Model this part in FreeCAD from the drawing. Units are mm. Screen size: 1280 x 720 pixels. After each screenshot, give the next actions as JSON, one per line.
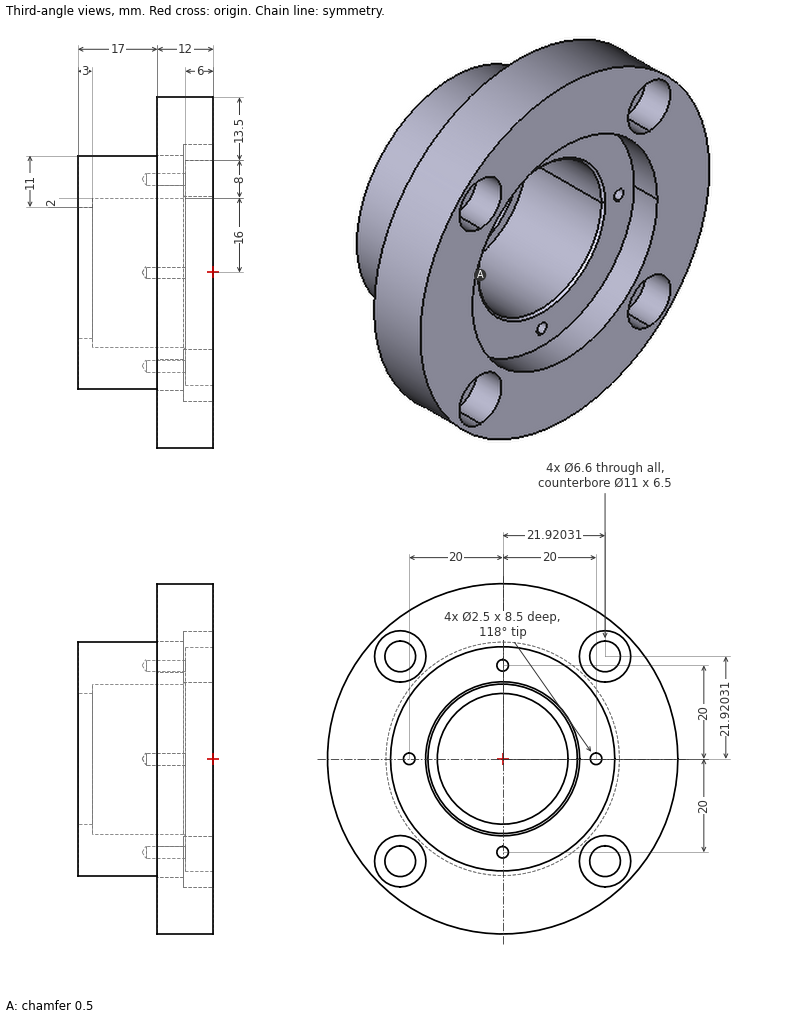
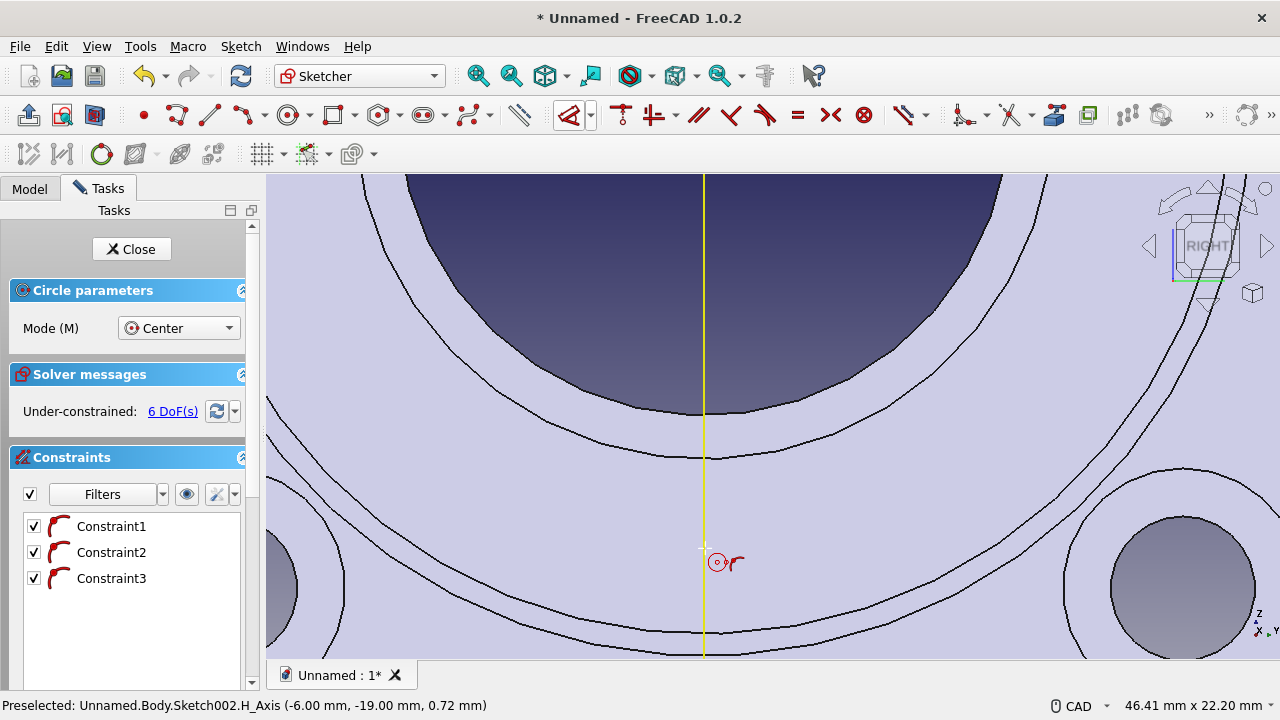
{"action": "left_click", "coordinate": [704, 547]}
{"action": "left_click", "coordinate": [723, 527]}
{"action": "key", "text": "Escape"}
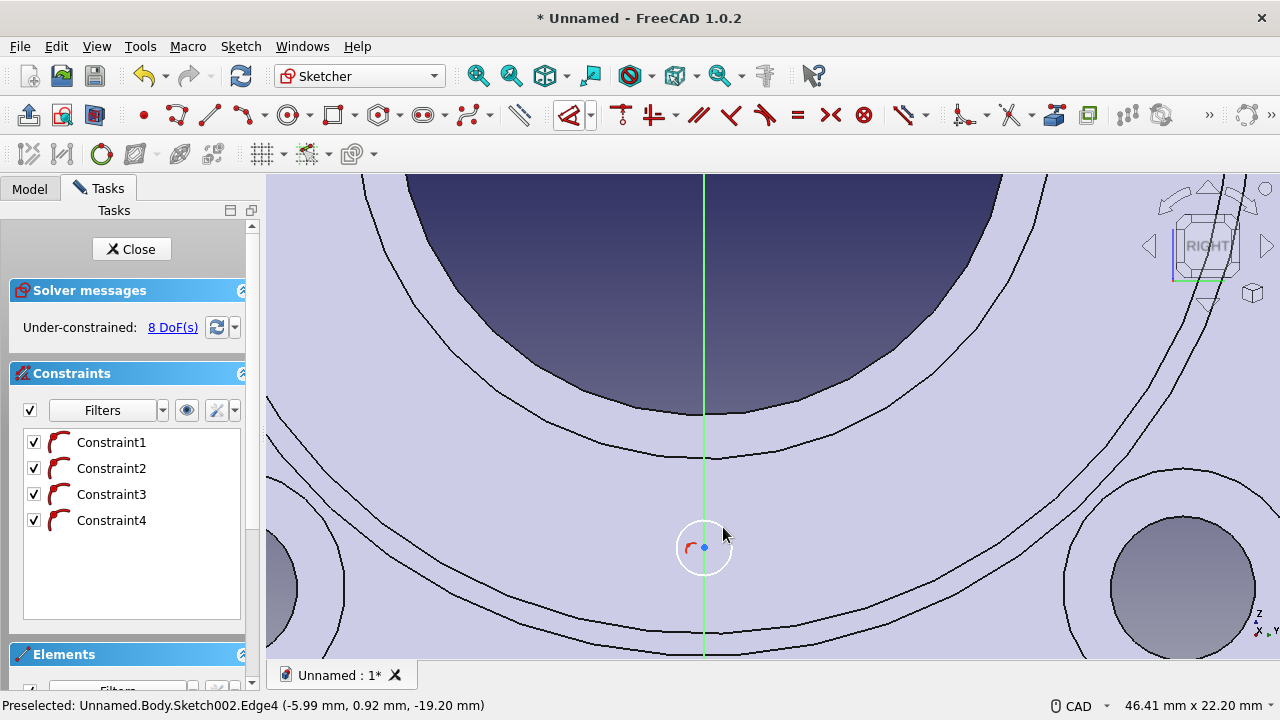
{"action": "scroll", "coordinate": [705, 549], "scroll_direction": "down", "scroll_amount": 6}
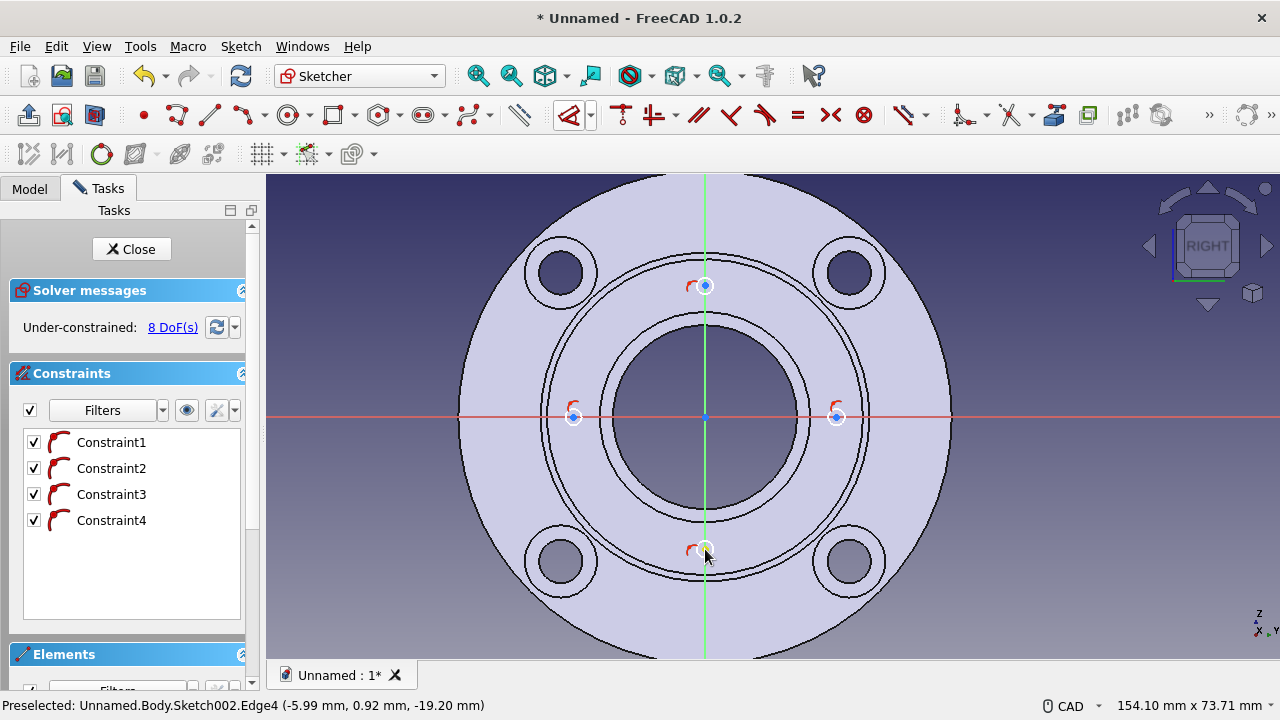
{"action": "scroll", "coordinate": [842, 411], "scroll_direction": "up", "scroll_amount": 5}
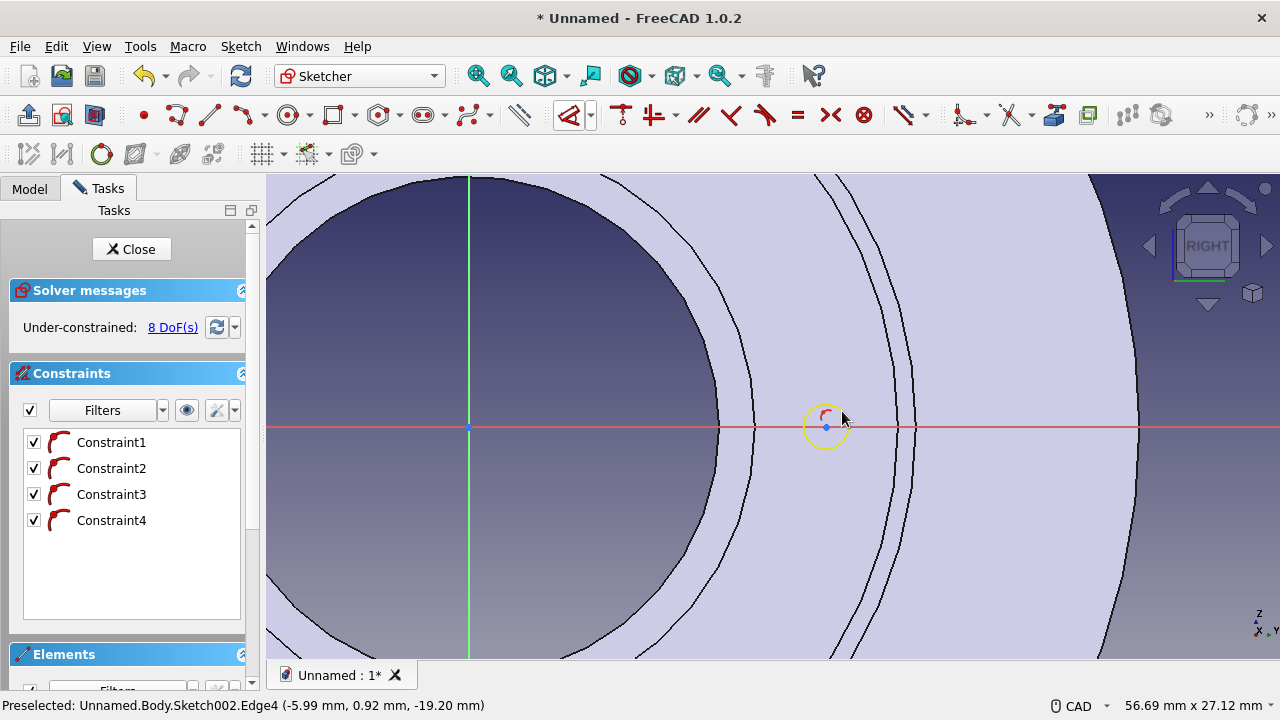
{"action": "left_click", "coordinate": [842, 411]}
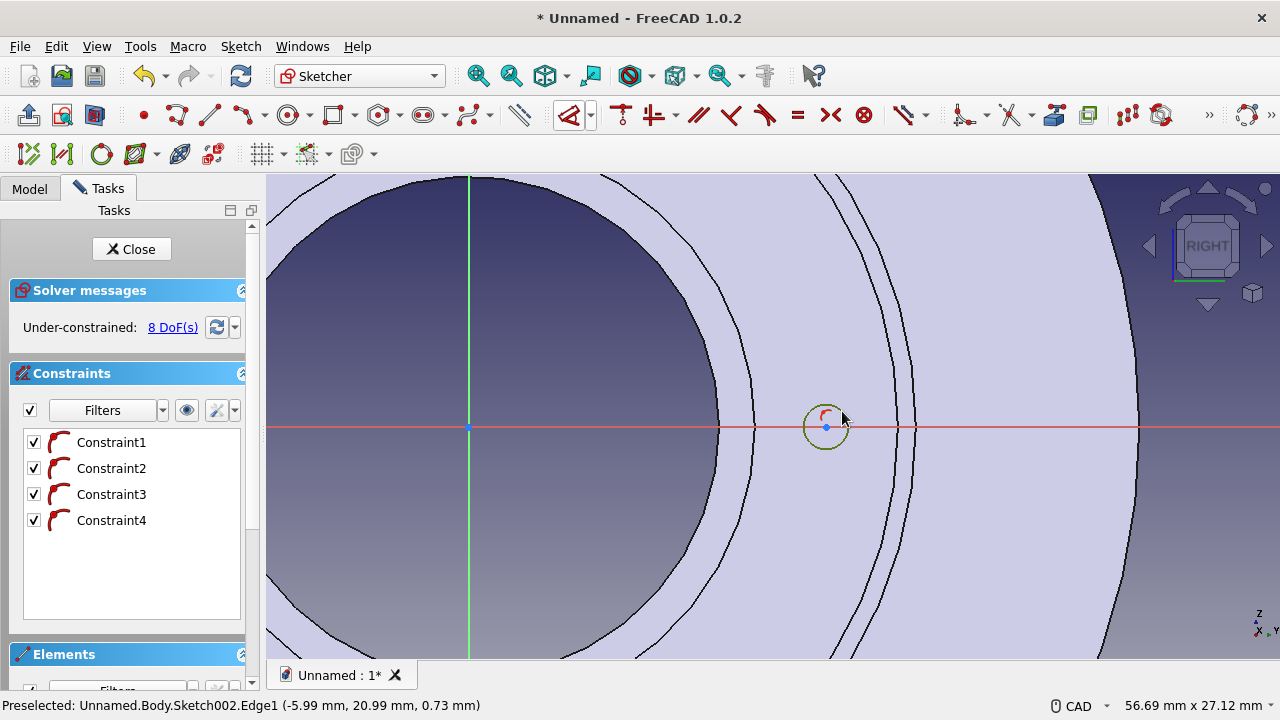
{"action": "scroll", "coordinate": [842, 410], "scroll_direction": "down", "scroll_amount": 5}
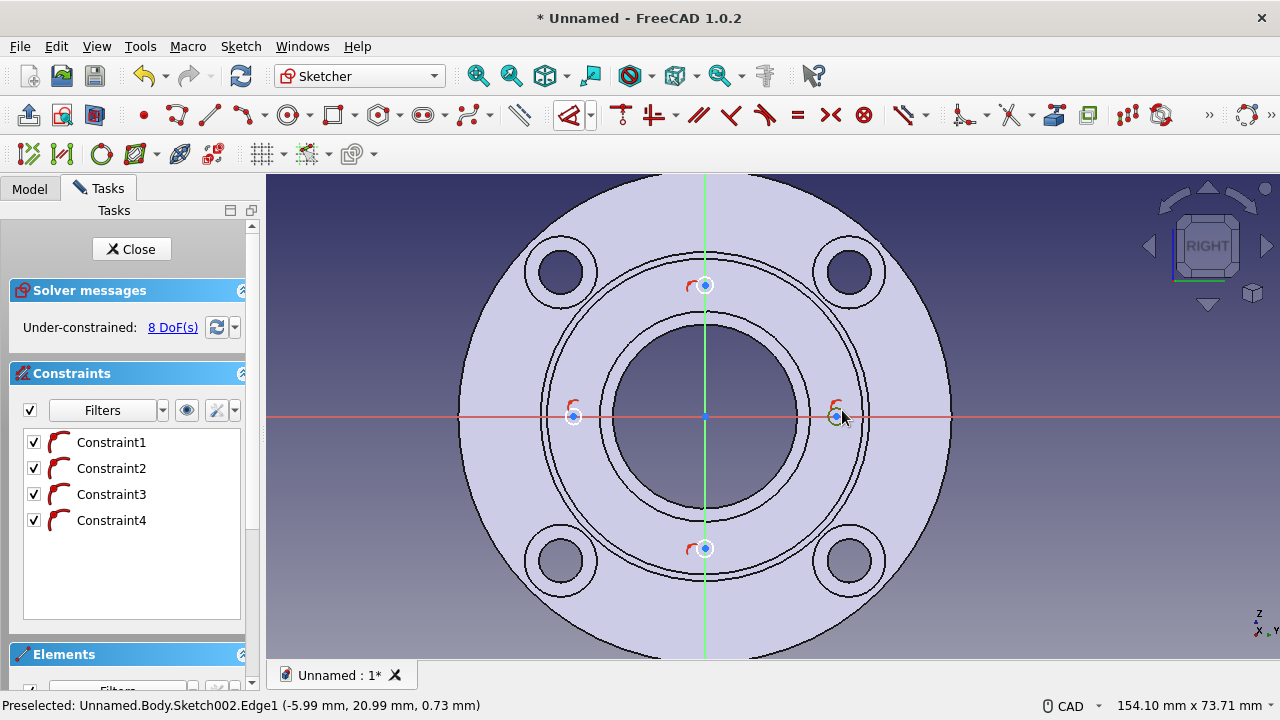
{"action": "scroll", "coordinate": [711, 279], "scroll_direction": "up", "scroll_amount": 5}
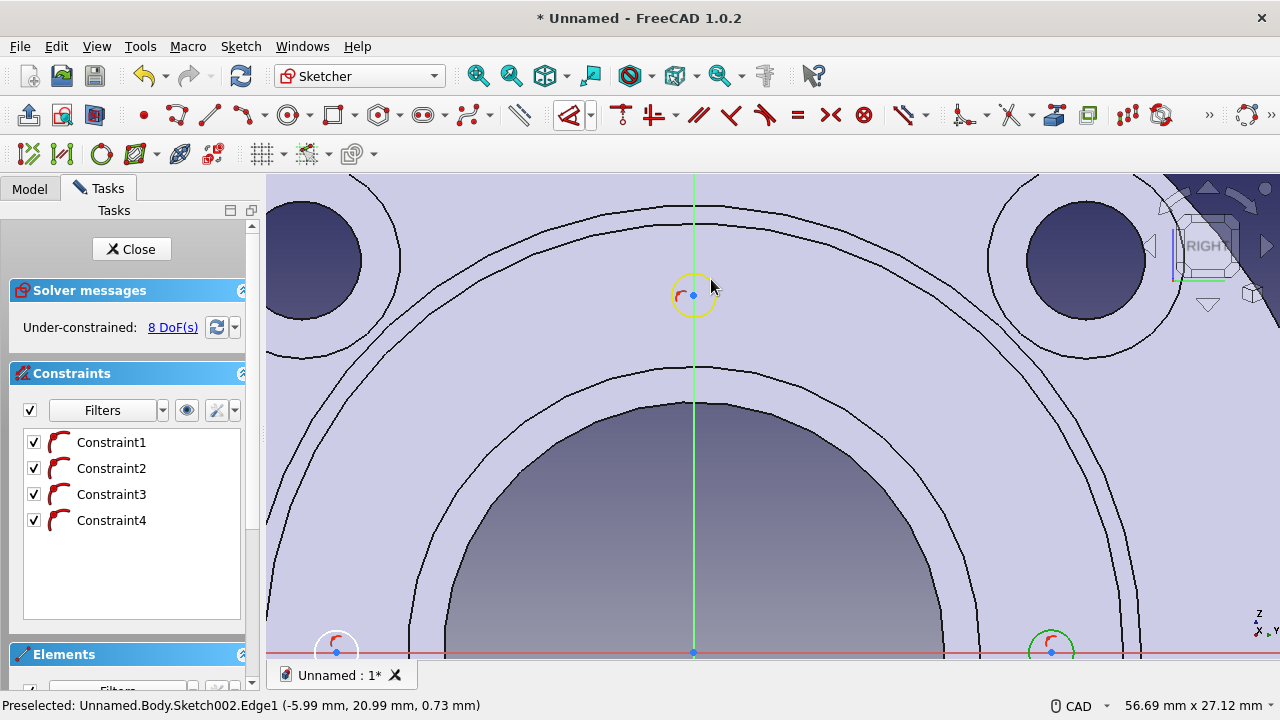
{"action": "left_click", "coordinate": [709, 280]}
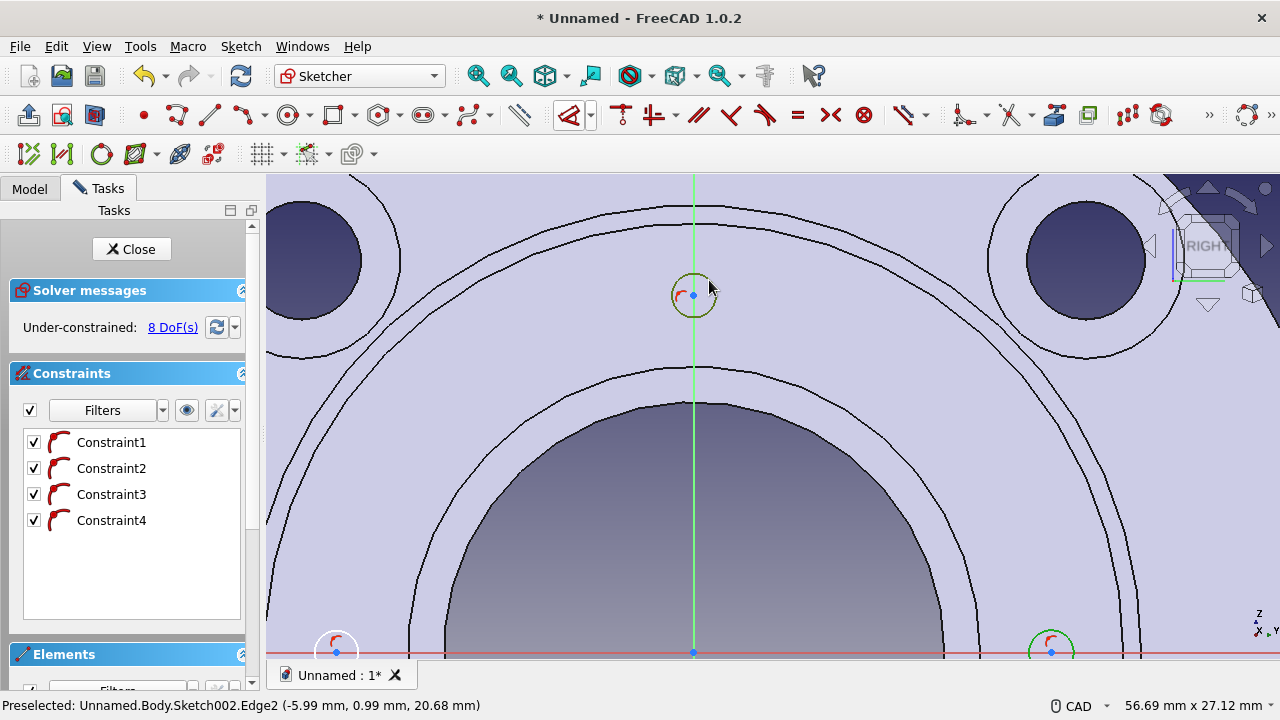
{"action": "left_click", "coordinate": [337, 631]}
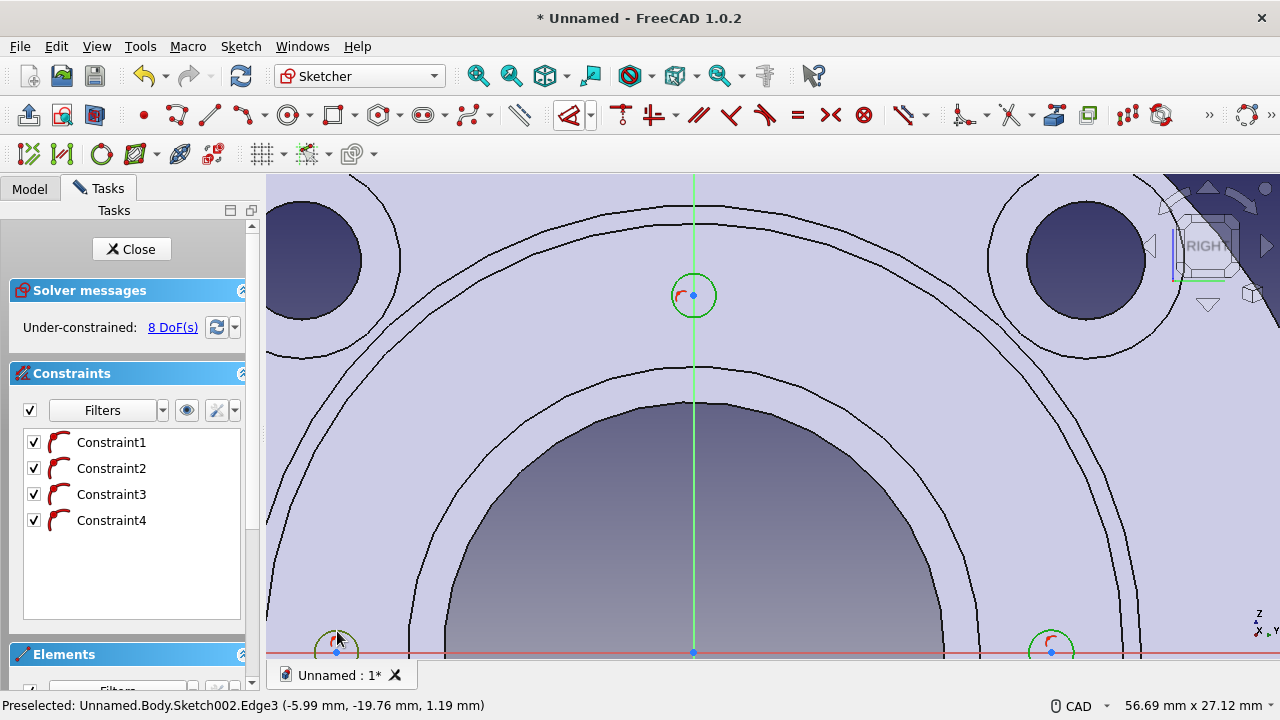
{"action": "scroll", "coordinate": [711, 279], "scroll_direction": "down", "scroll_amount": 5}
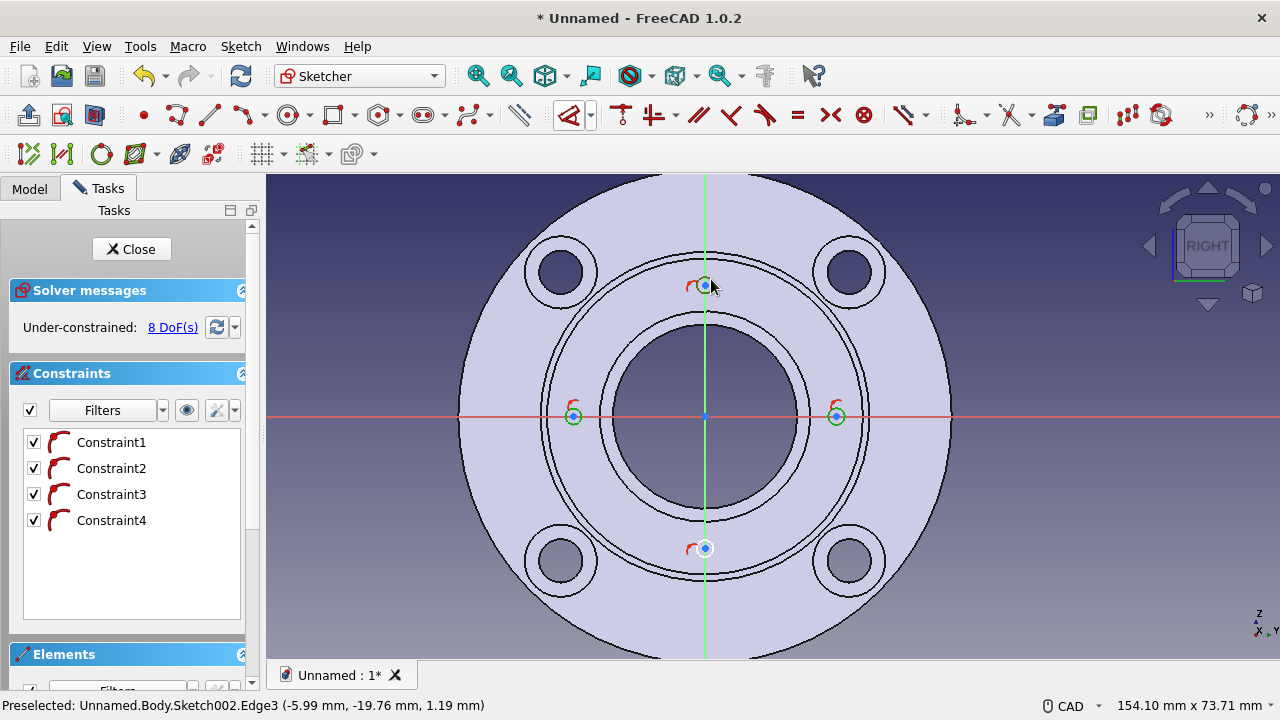
{"action": "scroll", "coordinate": [711, 543], "scroll_direction": "up", "scroll_amount": 5}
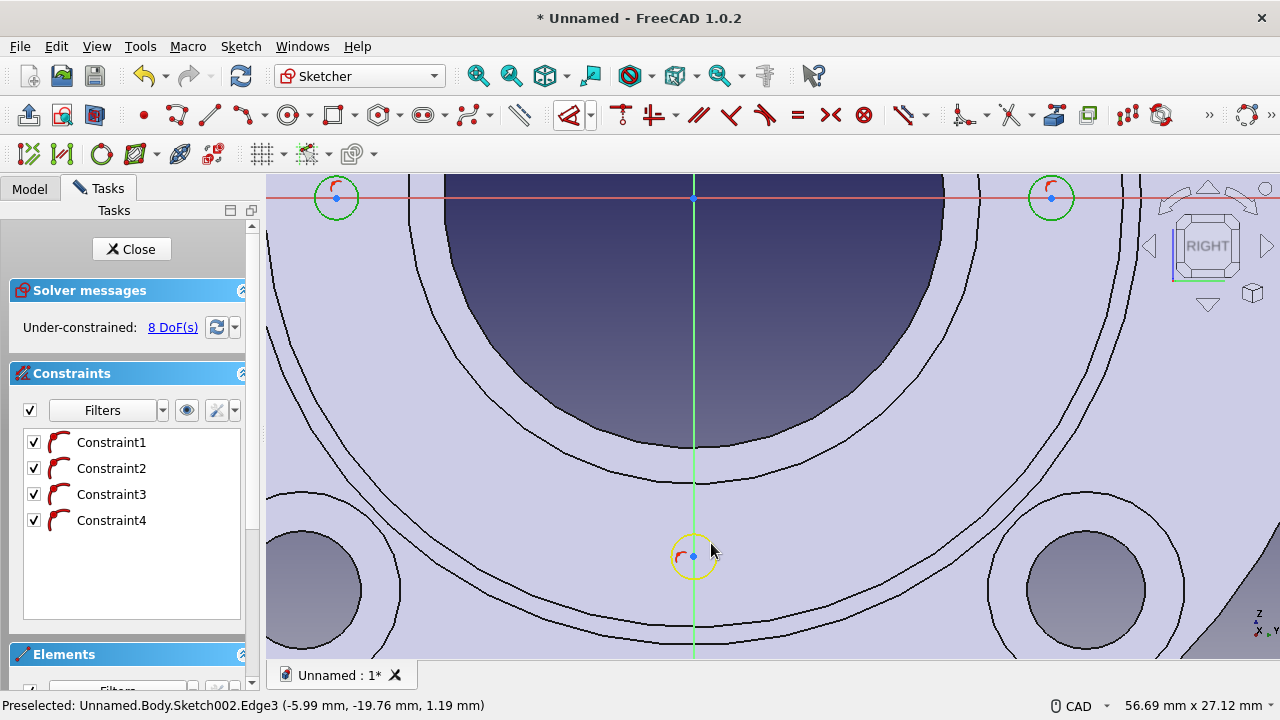
{"action": "left_click", "coordinate": [710, 541]}